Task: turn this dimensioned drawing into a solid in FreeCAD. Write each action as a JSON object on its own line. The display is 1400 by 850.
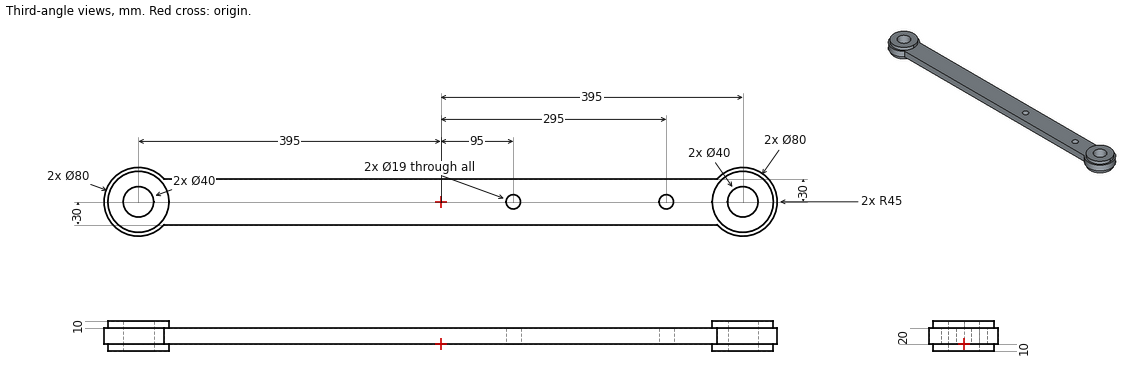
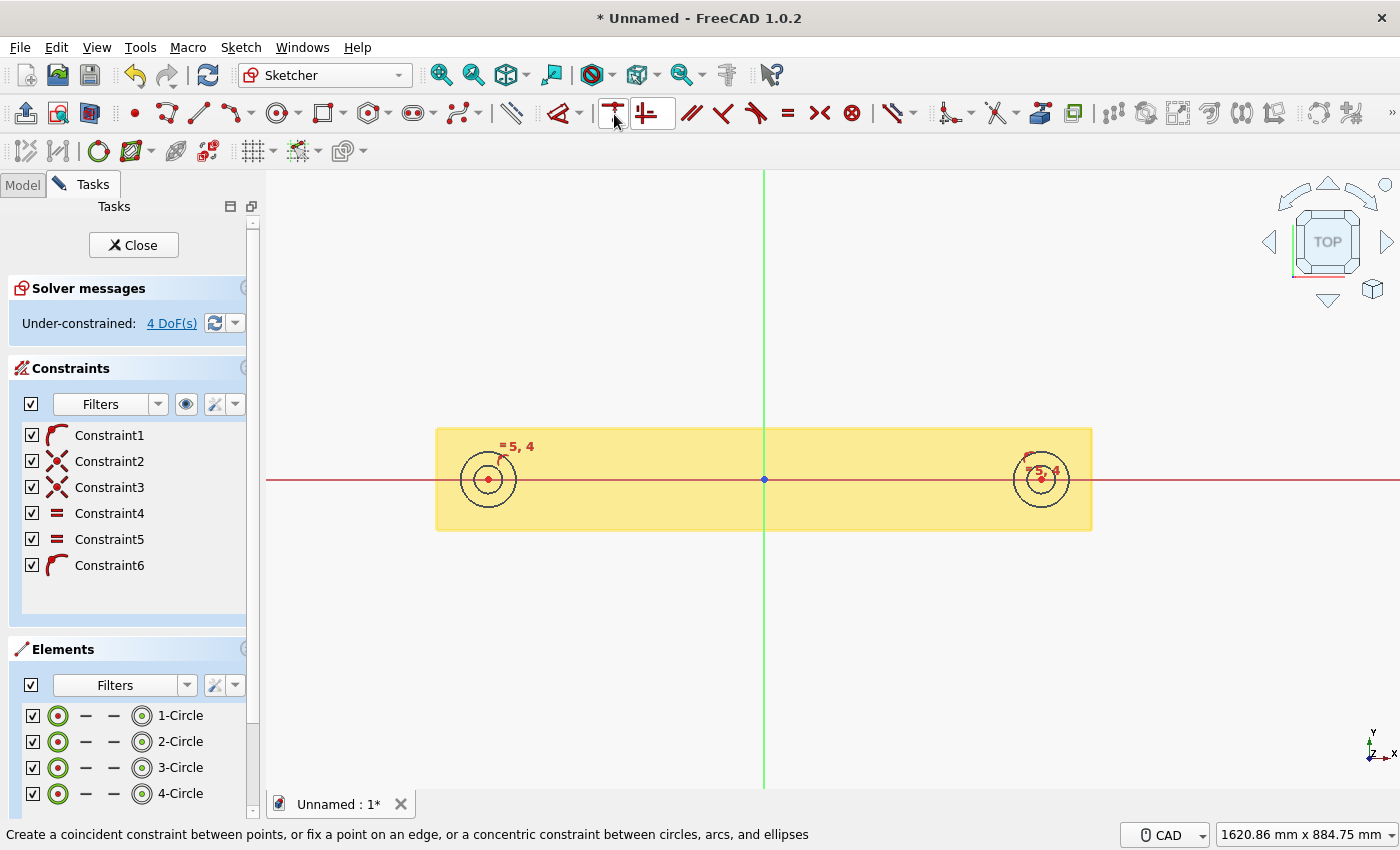
{"action": "left_click", "coordinate": [558, 114]}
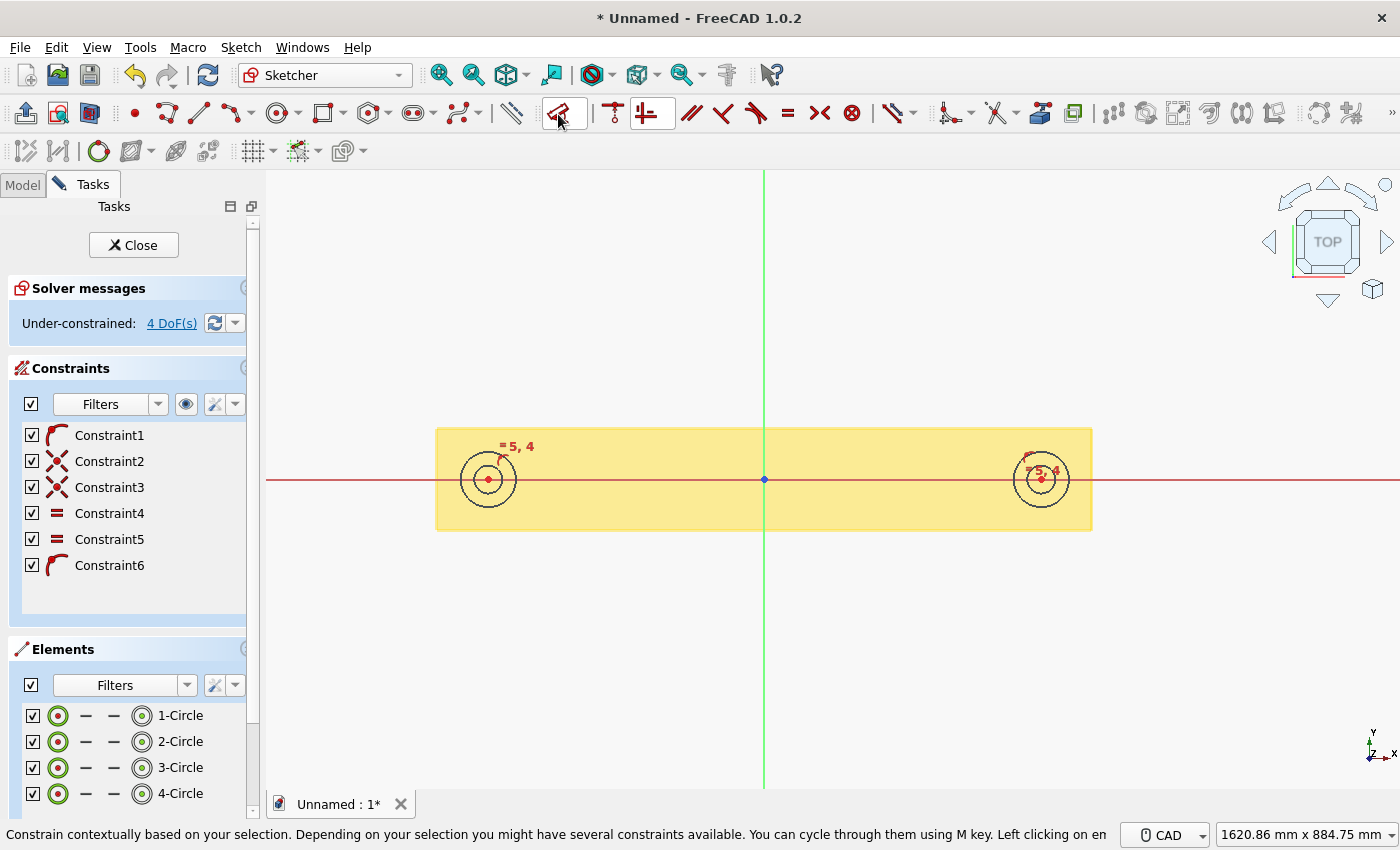
{"action": "left_click", "coordinate": [1061, 460]}
{"action": "left_click", "coordinate": [1084, 437]}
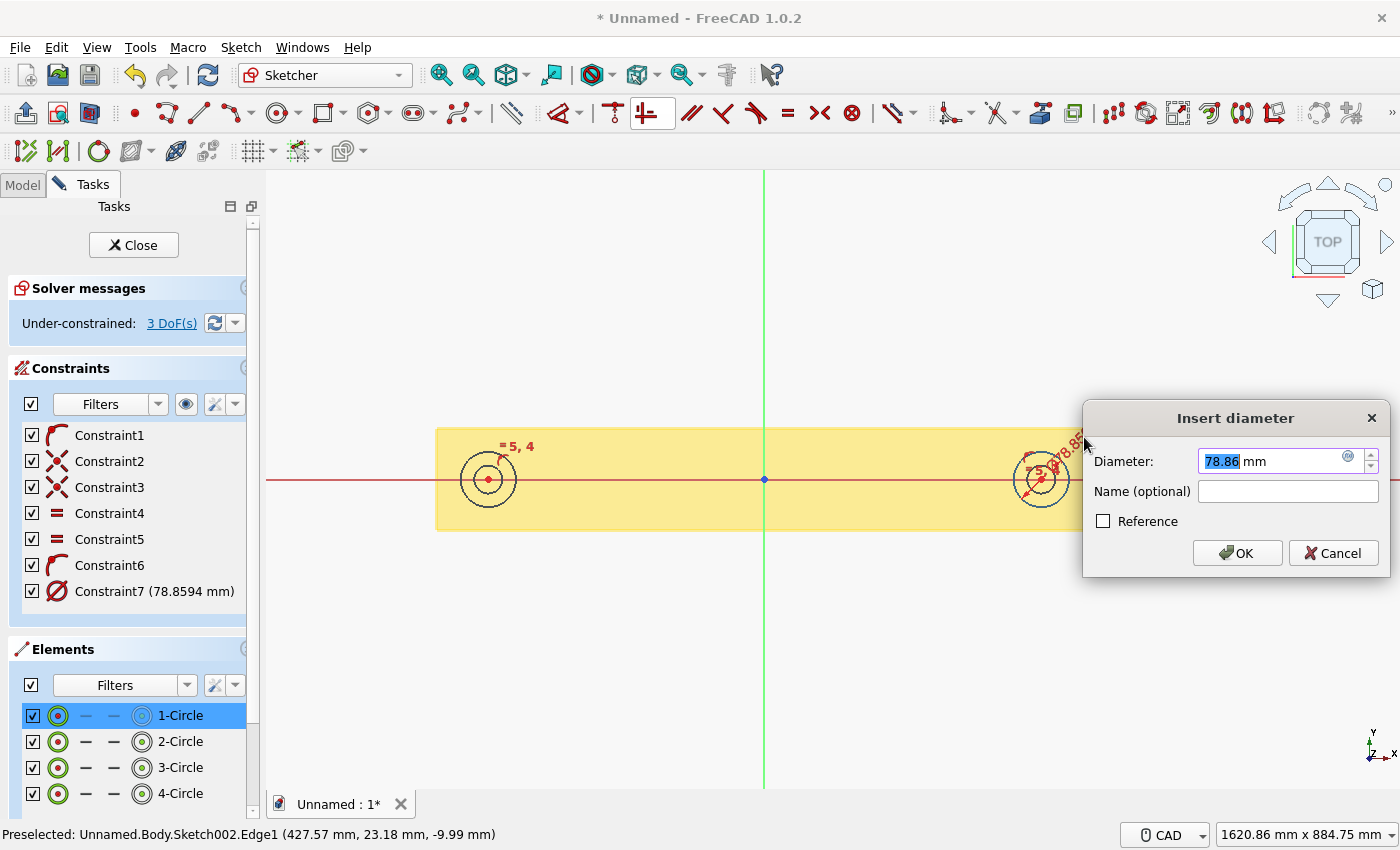
{"action": "type", "text": "80"}
{"action": "key", "text": "Return"}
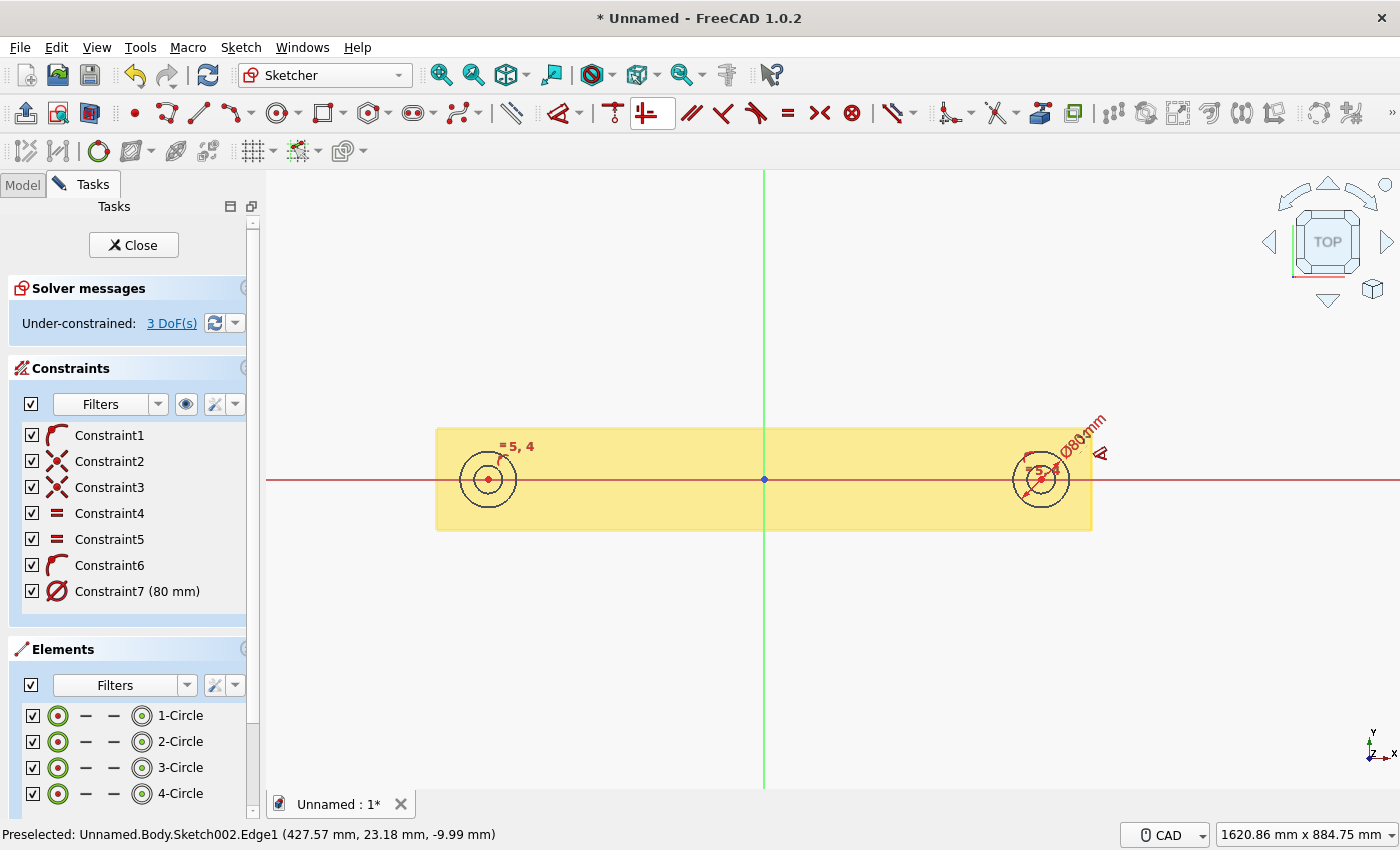
{"action": "scroll", "coordinate": [1051, 470], "scroll_direction": "up", "scroll_amount": 2}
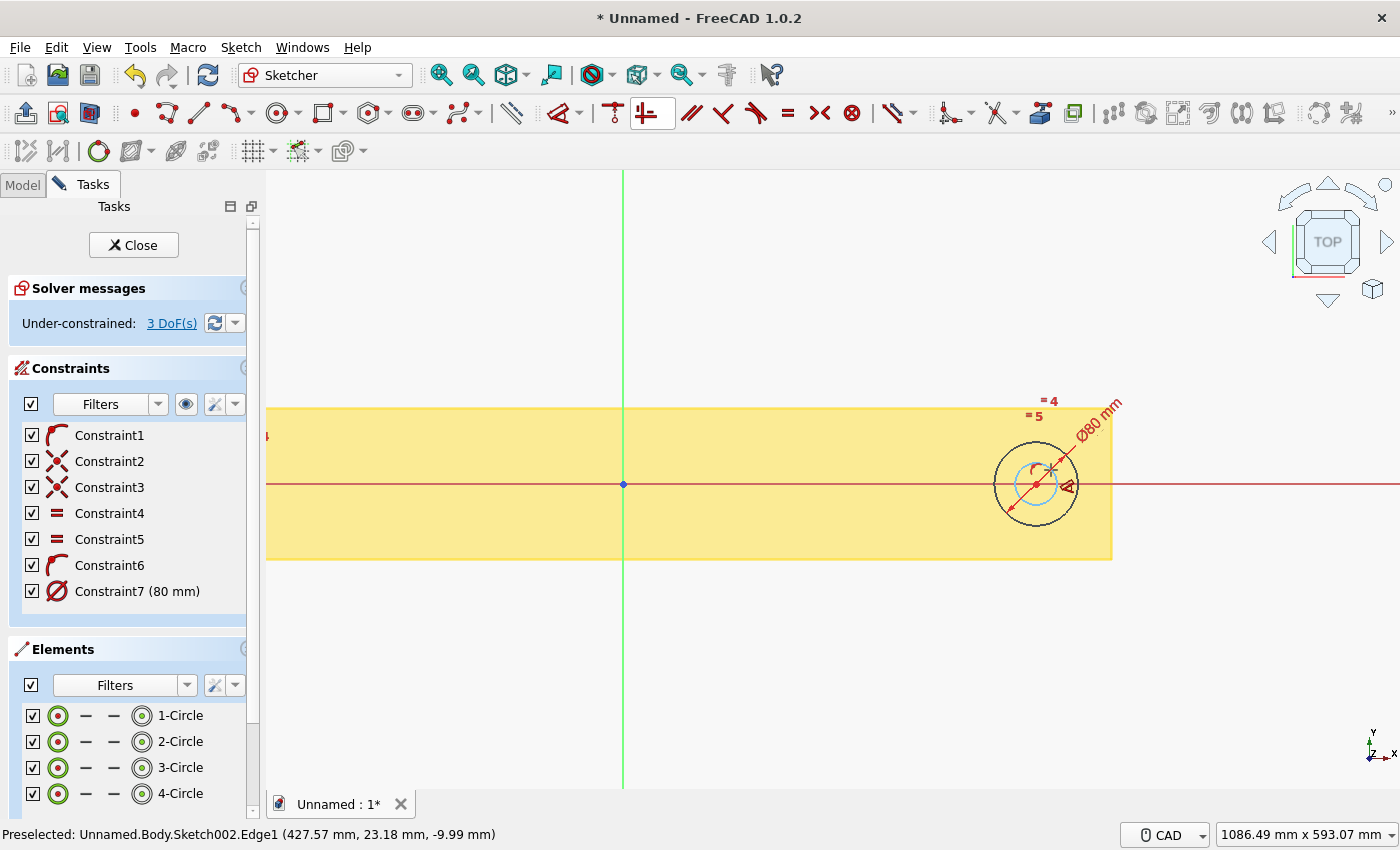
{"action": "left_click", "coordinate": [1051, 469]}
{"action": "left_click", "coordinate": [1109, 462]}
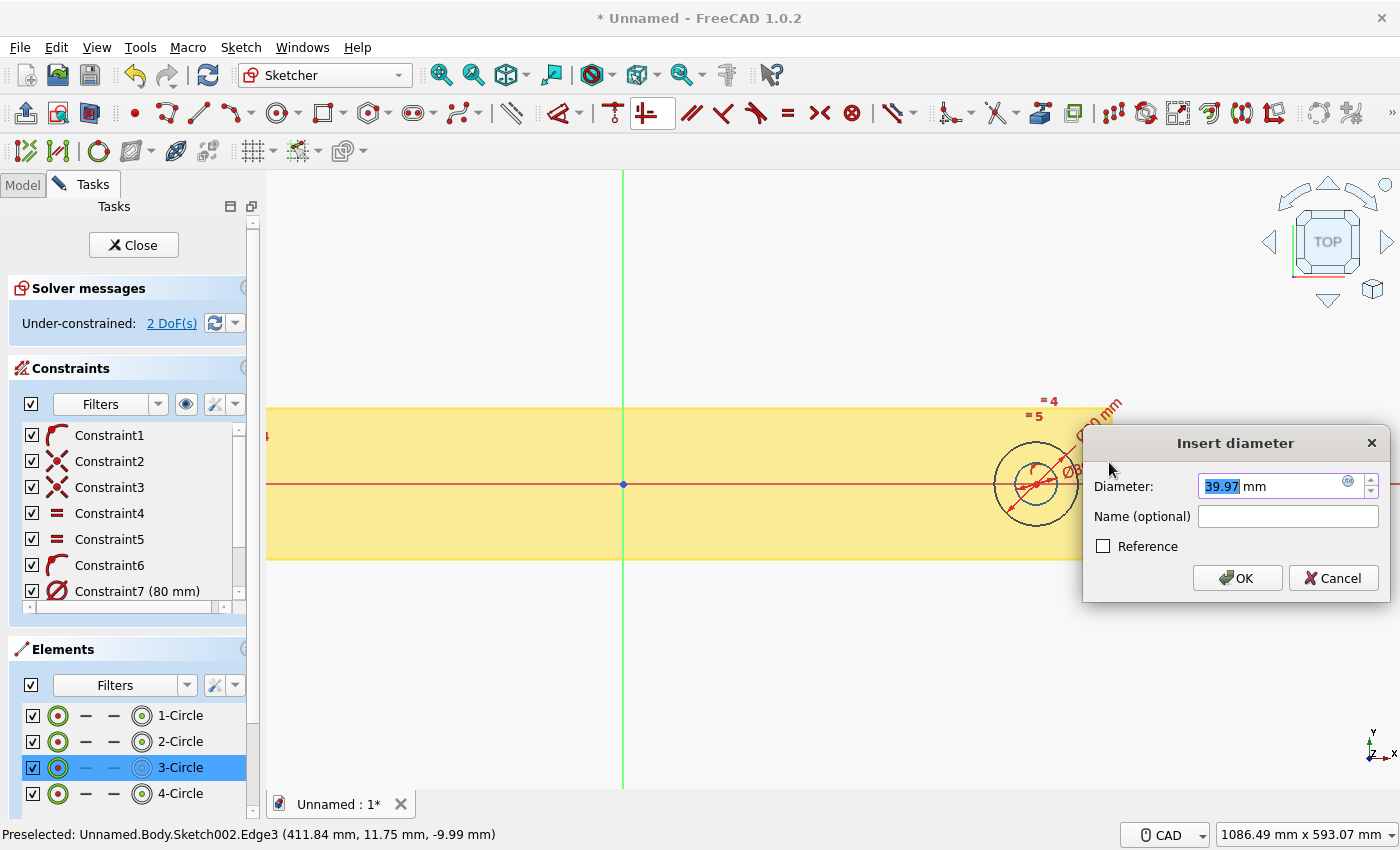
{"action": "type", "text": "40"}
{"action": "key", "text": "Return"}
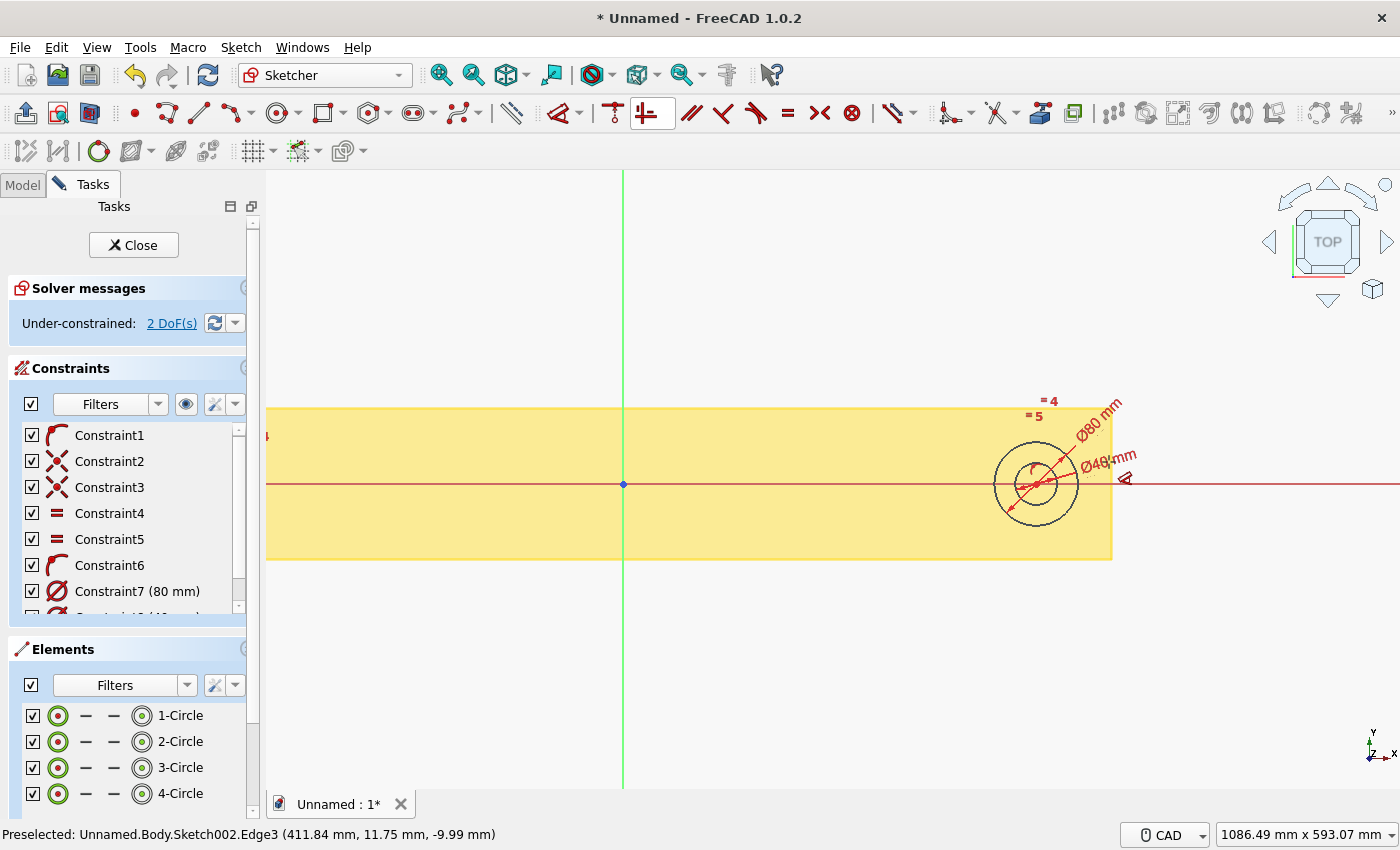
{"action": "left_click", "coordinate": [1036, 484]}
{"action": "left_click", "coordinate": [830, 518]}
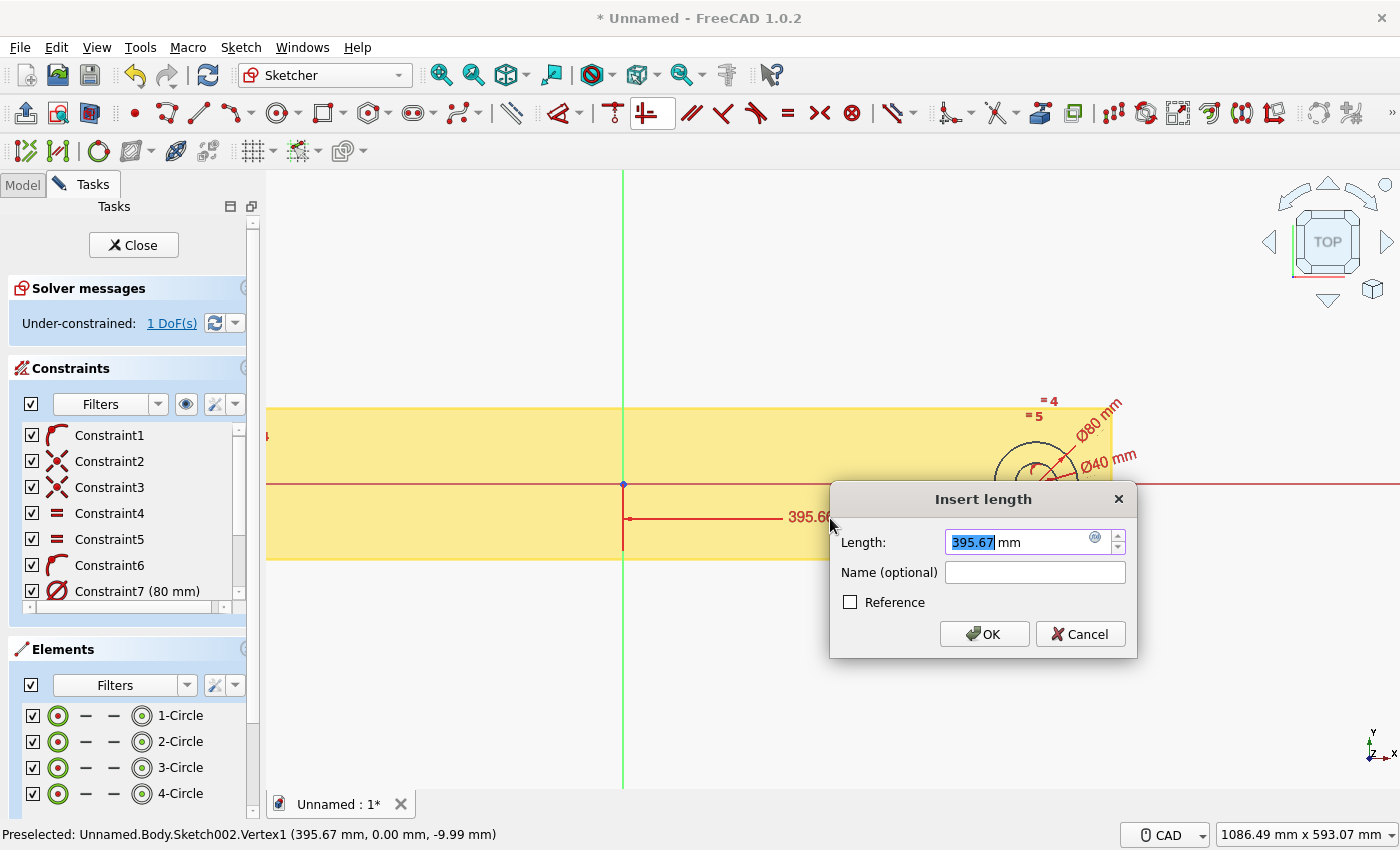
{"action": "type", "text": "395"}
{"action": "key", "text": "Return"}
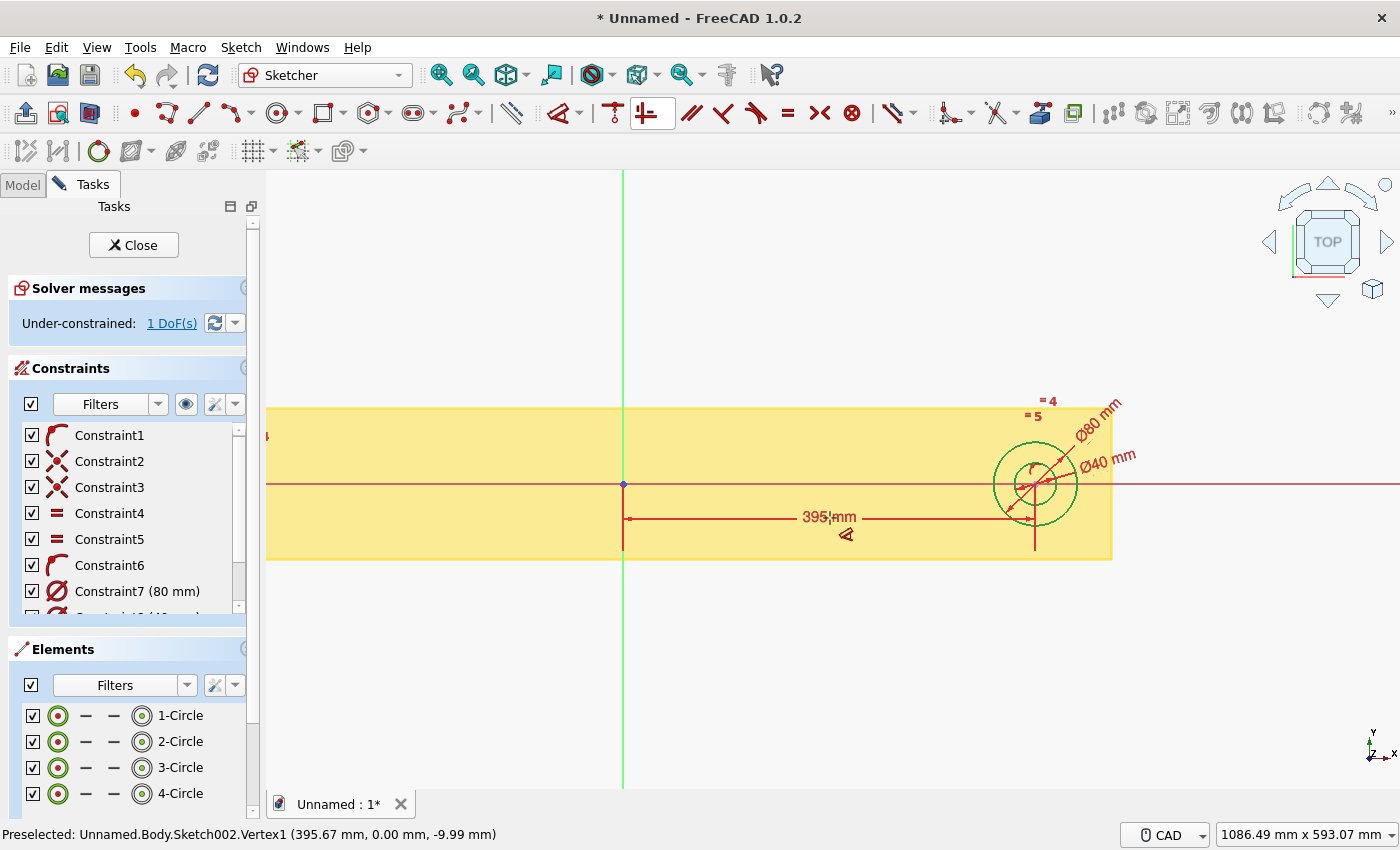
{"action": "scroll", "coordinate": [1052, 470], "scroll_direction": "down", "scroll_amount": 2}